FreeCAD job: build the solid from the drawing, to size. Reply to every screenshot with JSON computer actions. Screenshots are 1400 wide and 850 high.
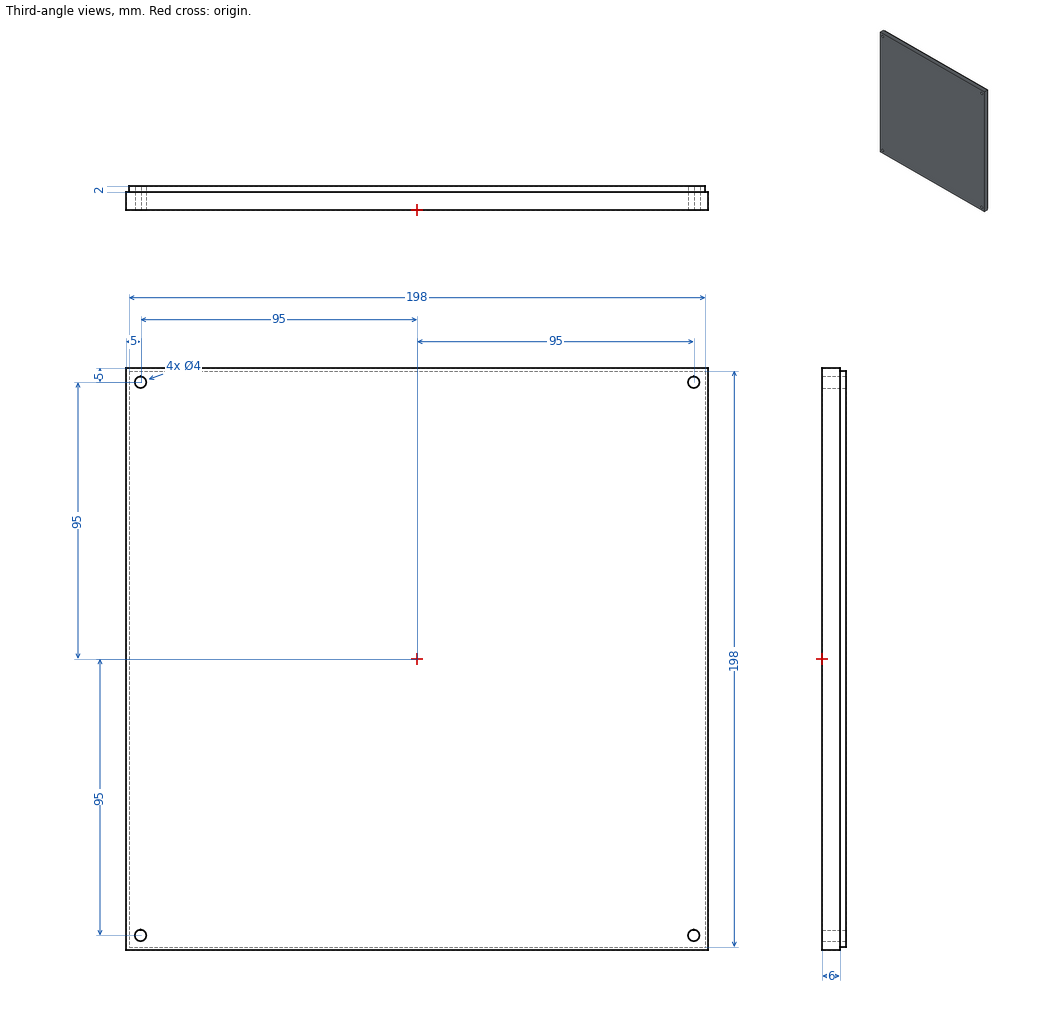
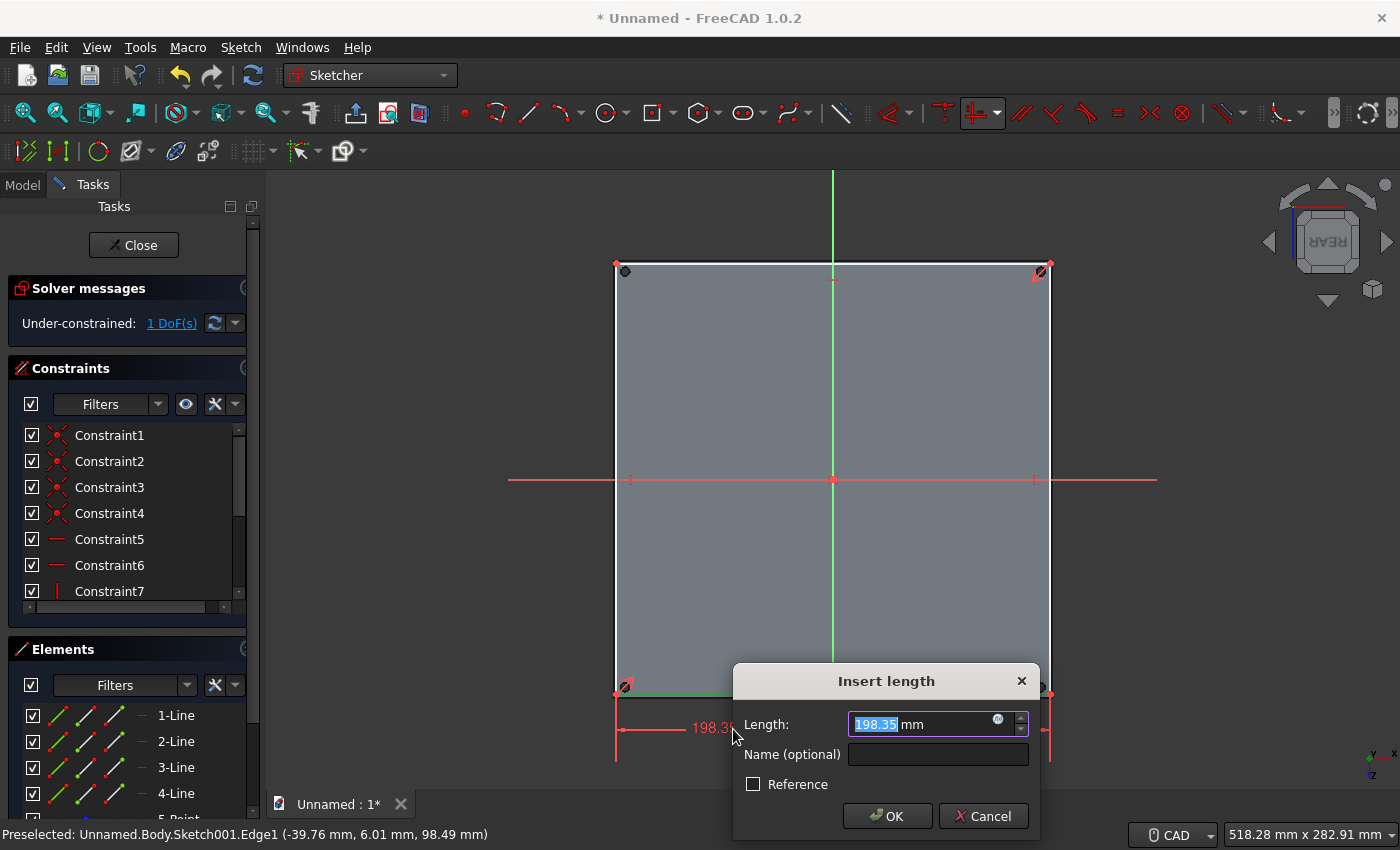
{"action": "type", "text": "198"}
{"action": "key", "text": "Return"}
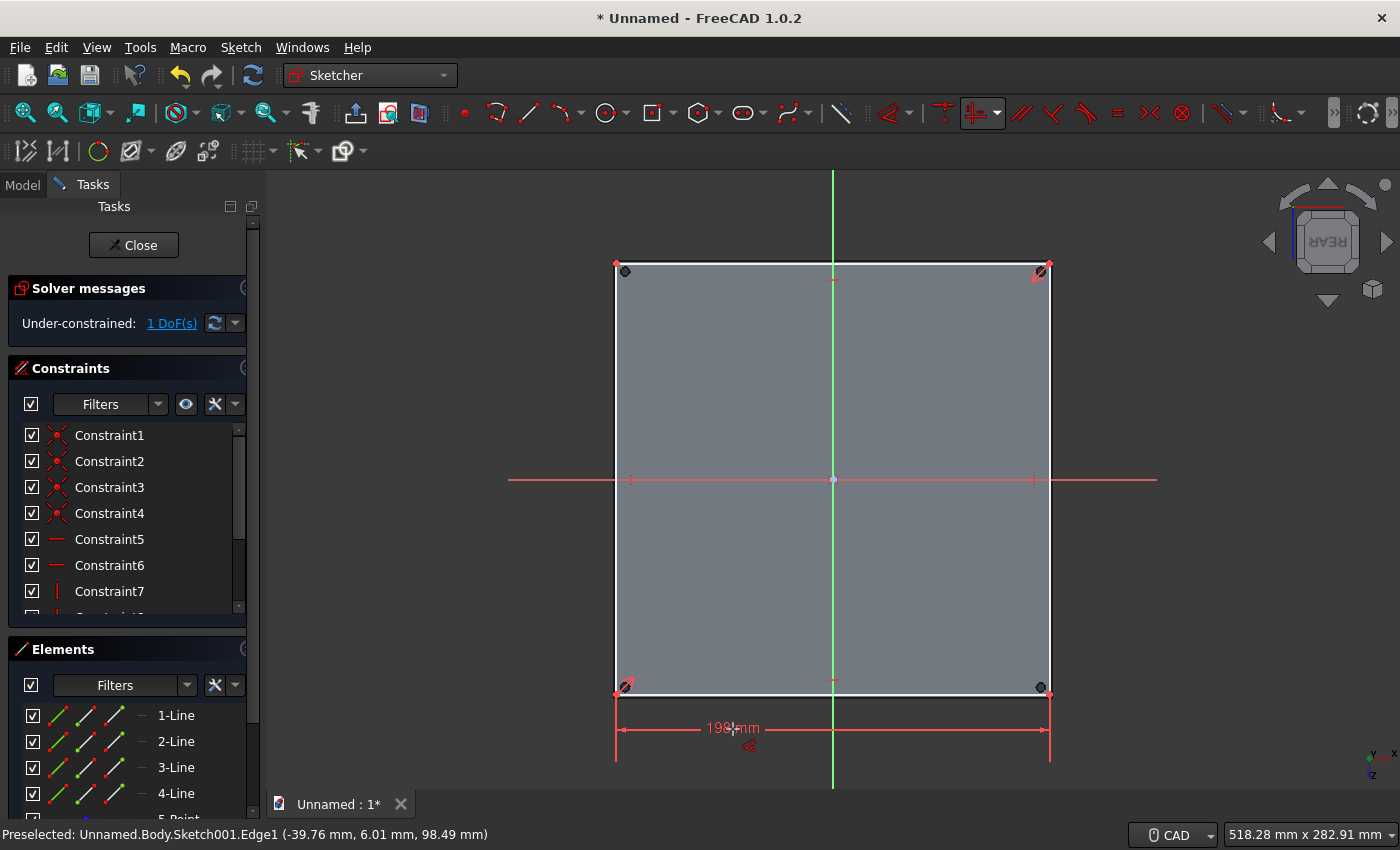
{"action": "left_click", "coordinate": [1050, 566]}
{"action": "left_click", "coordinate": [1084, 380]}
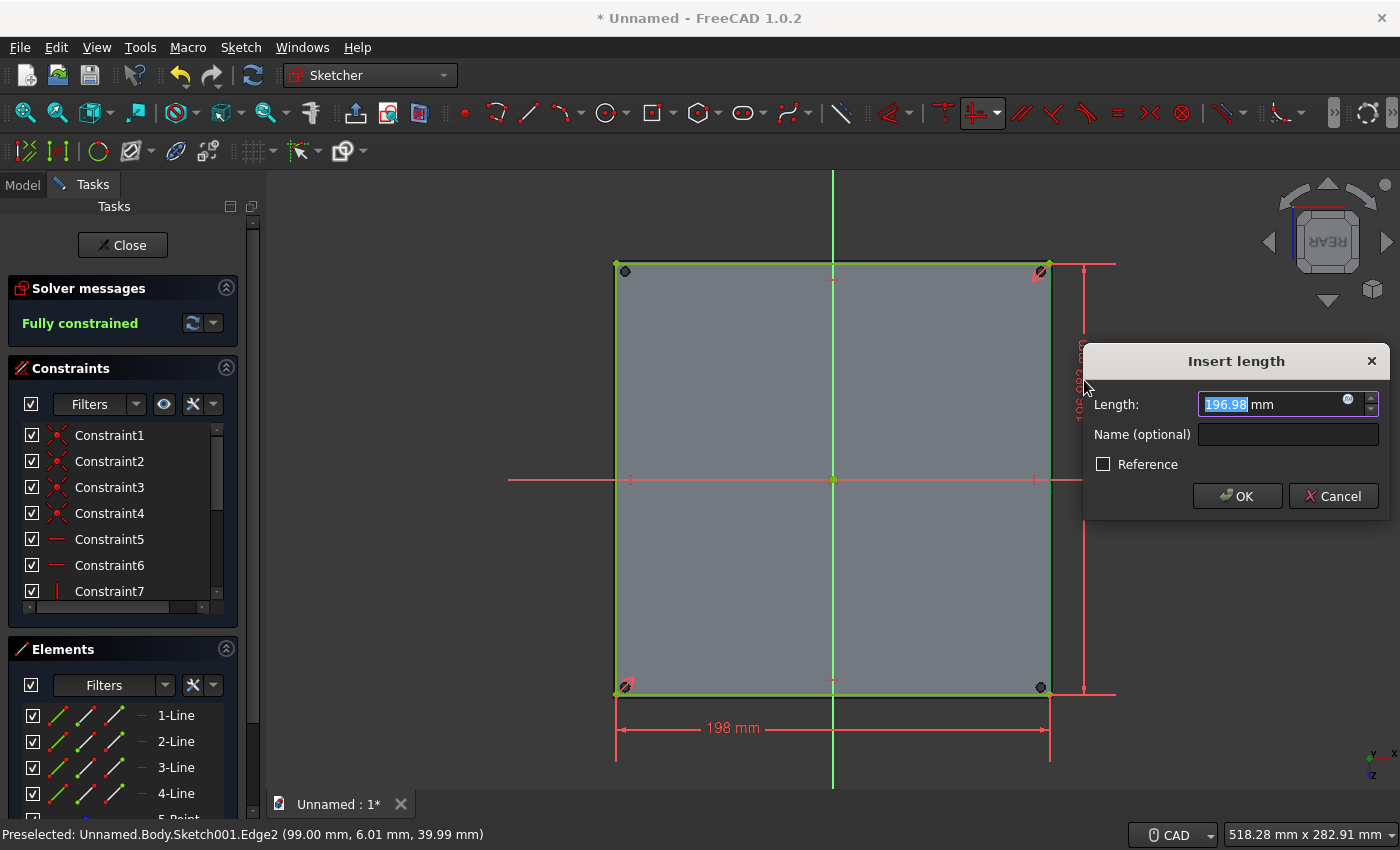
{"action": "type", "text": "198"}
{"action": "key", "text": "Return"}
{"action": "key", "text": "Escape"}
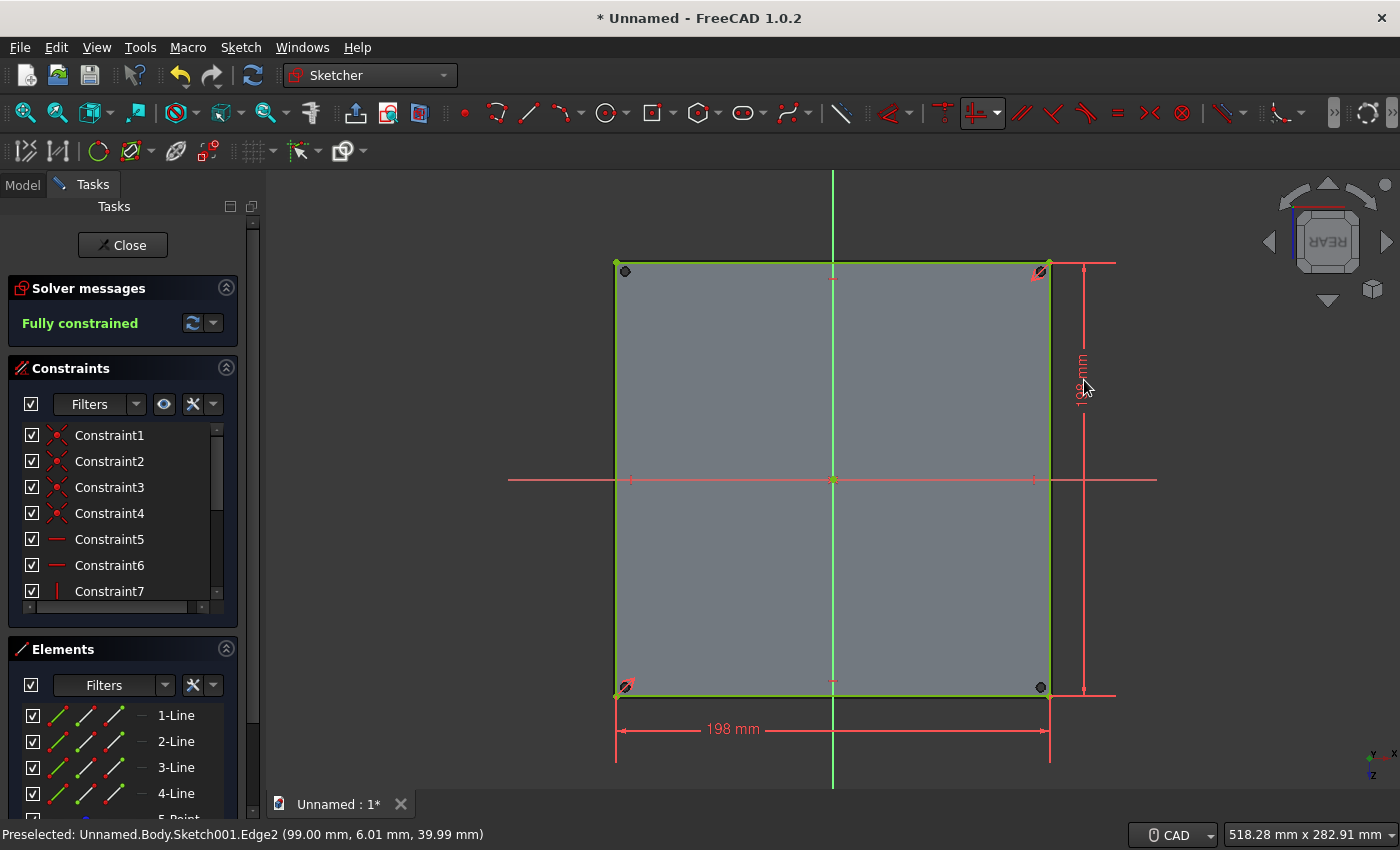
{"action": "left_click", "coordinate": [123, 245]}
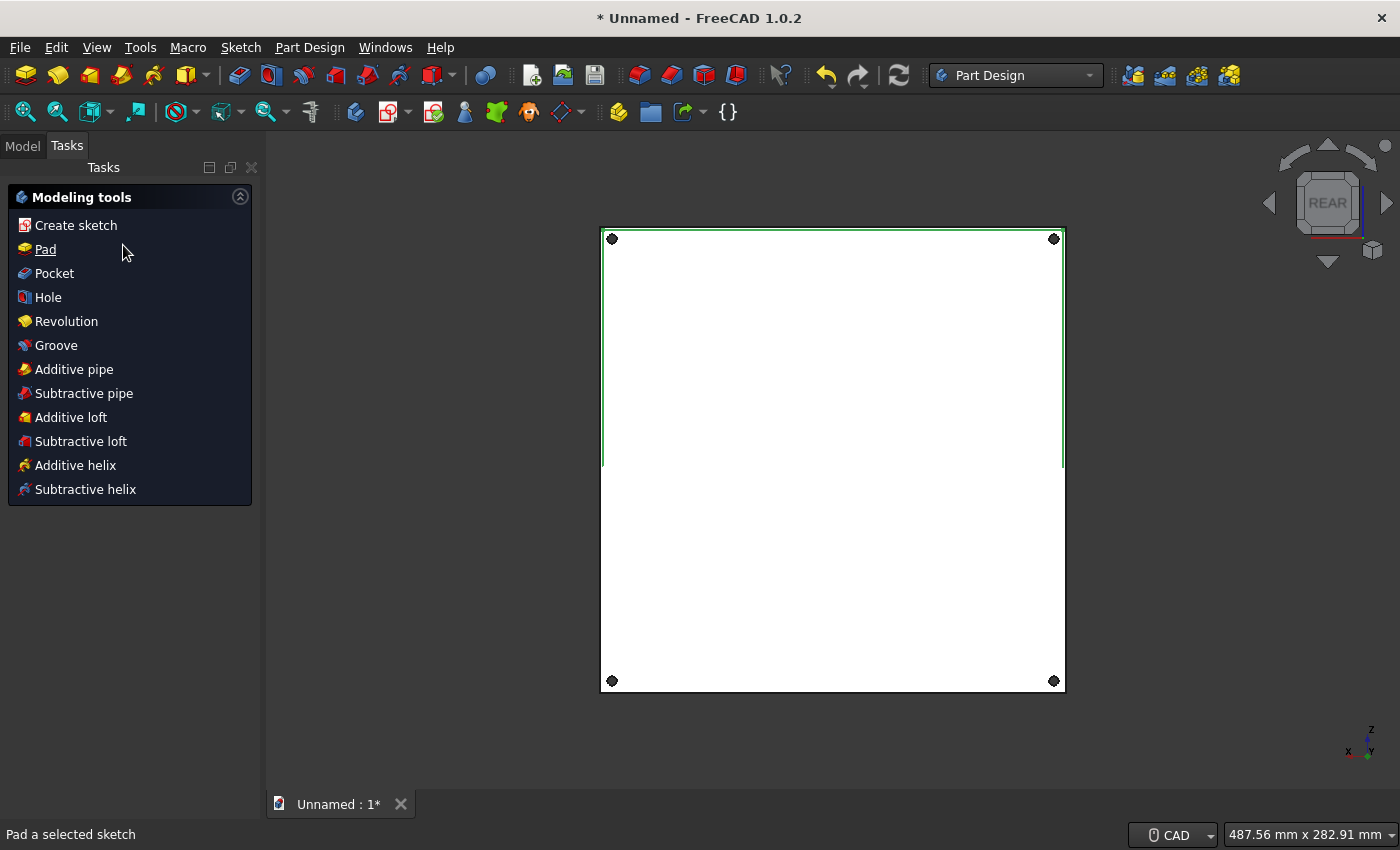
{"action": "left_click", "coordinate": [26, 76]}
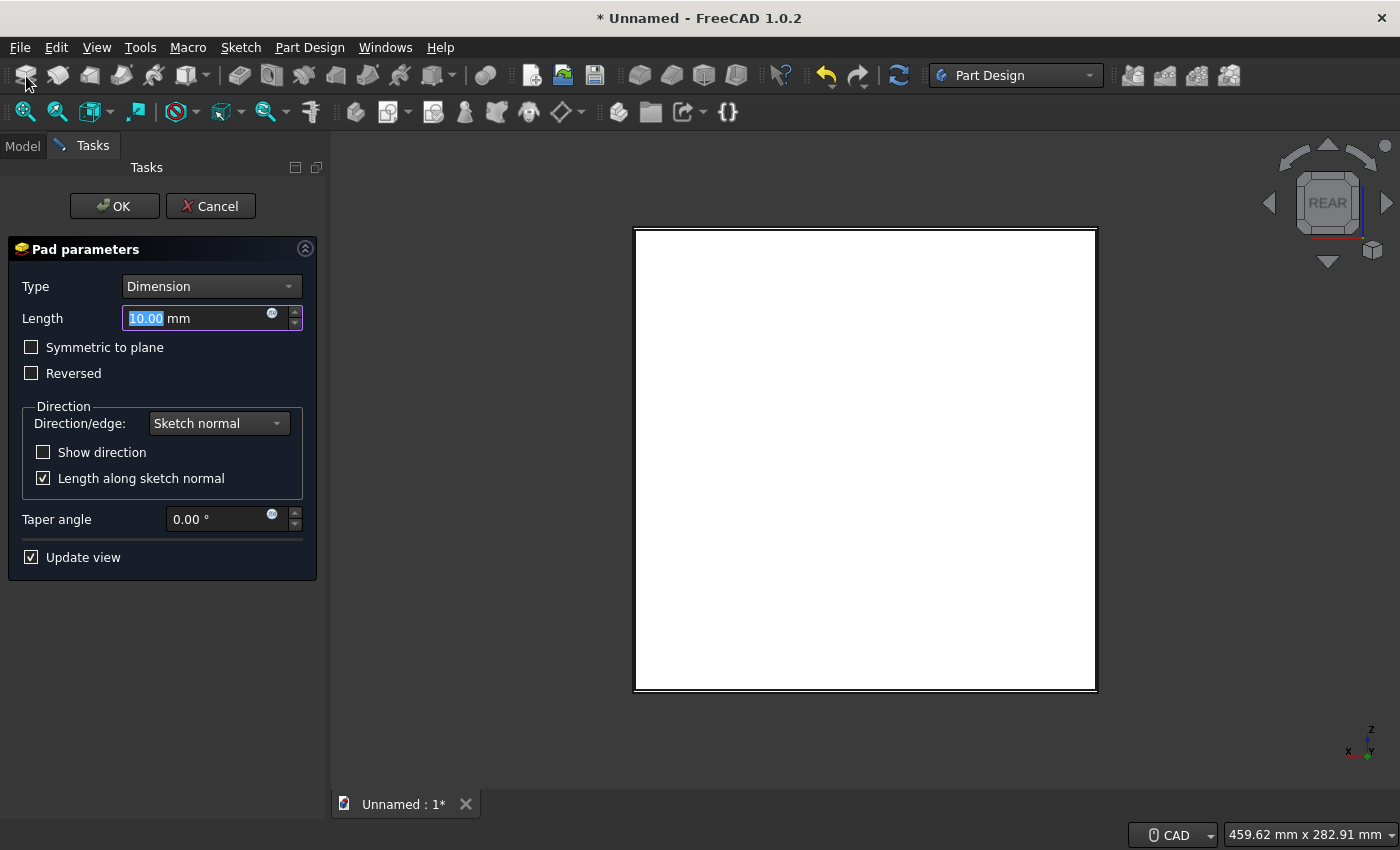
{"action": "type", "text": "2"}
{"action": "key", "text": "Tab"}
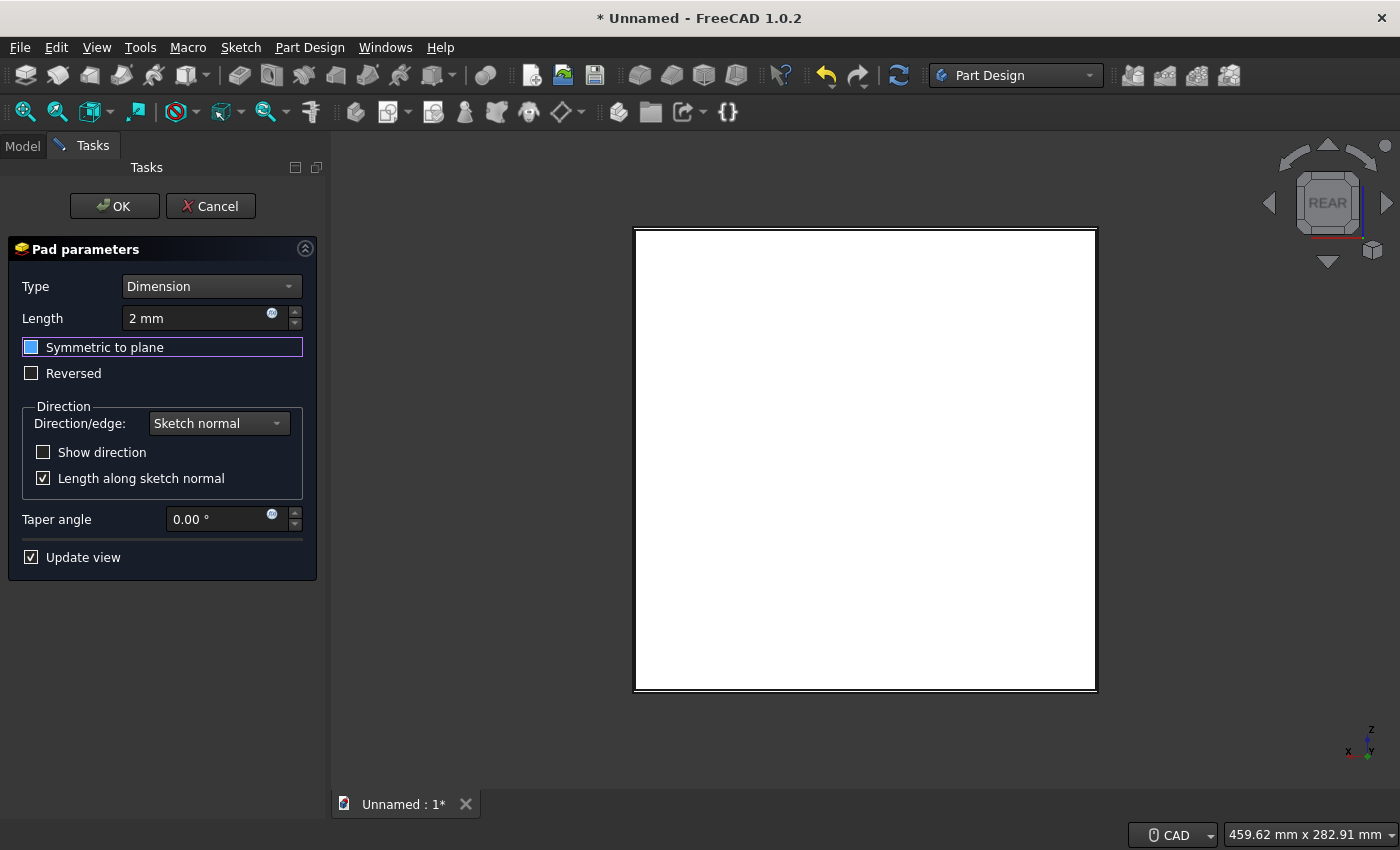
{"action": "left_click", "coordinate": [115, 206]}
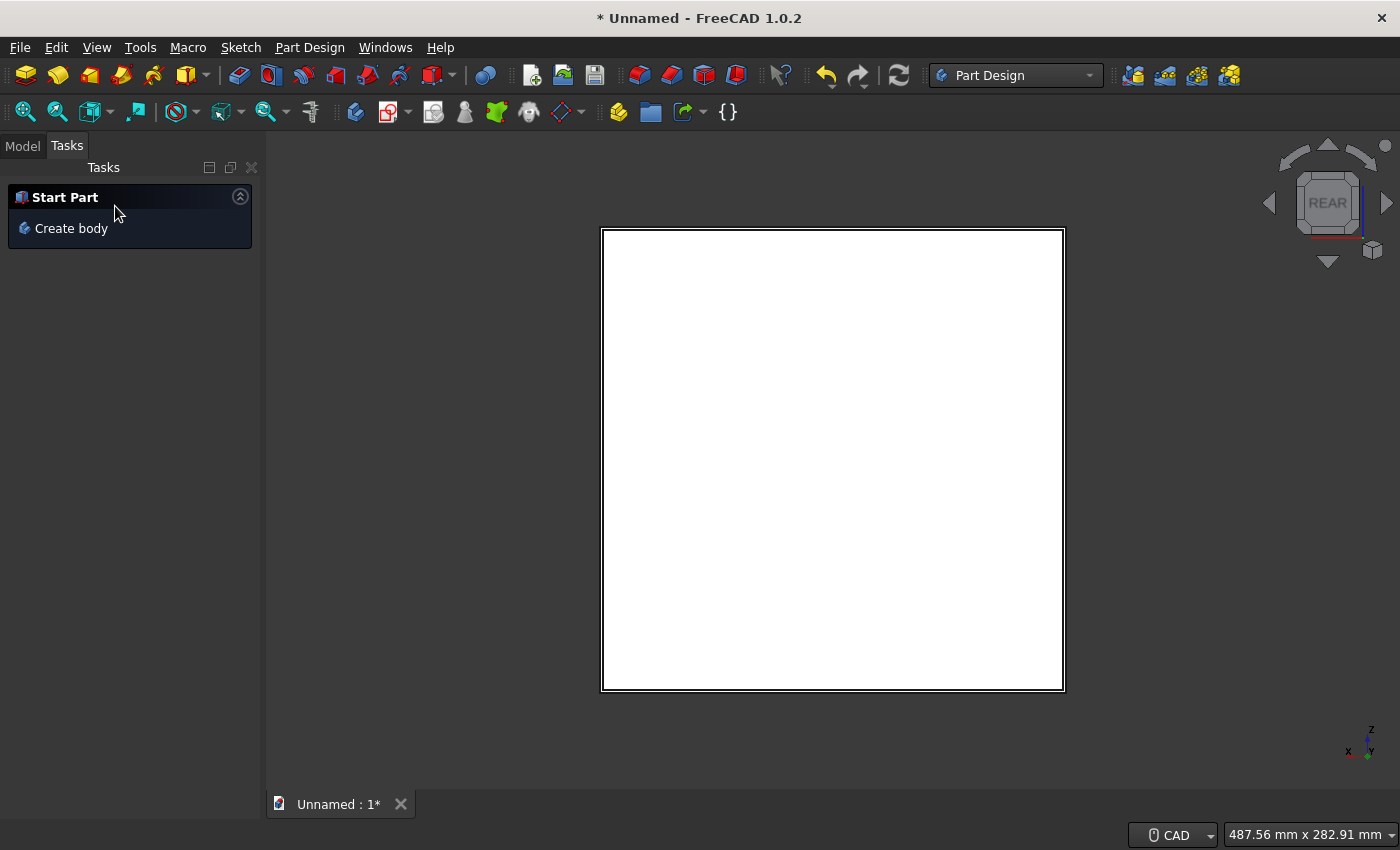
{"action": "left_click", "coordinate": [833, 459]}